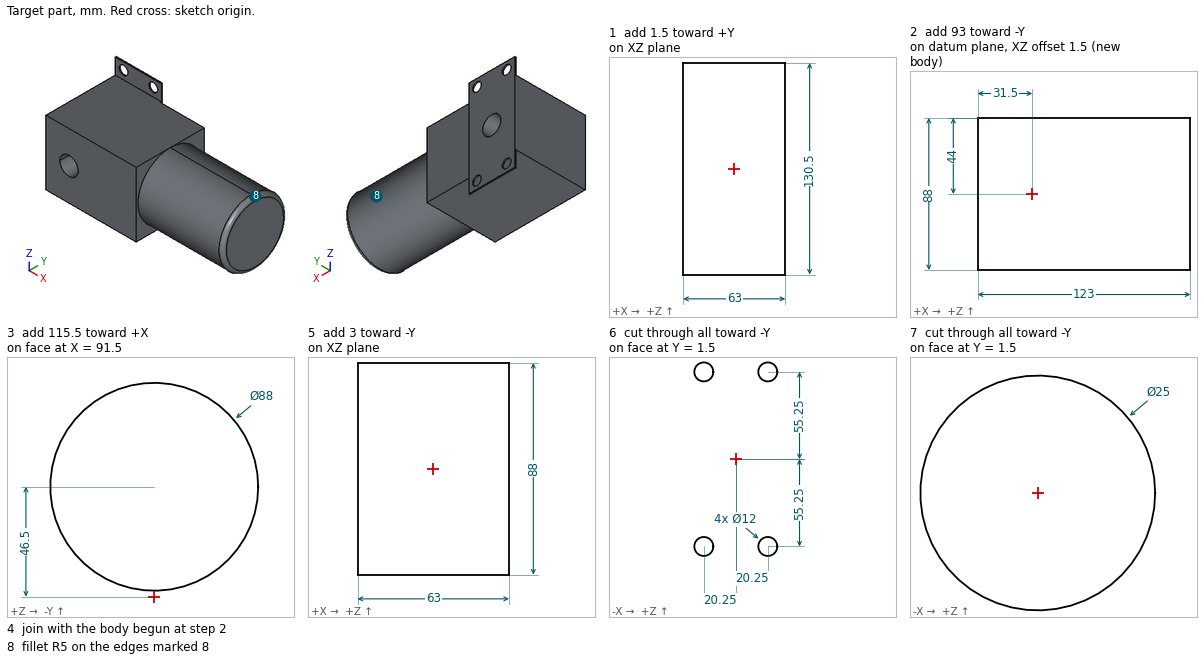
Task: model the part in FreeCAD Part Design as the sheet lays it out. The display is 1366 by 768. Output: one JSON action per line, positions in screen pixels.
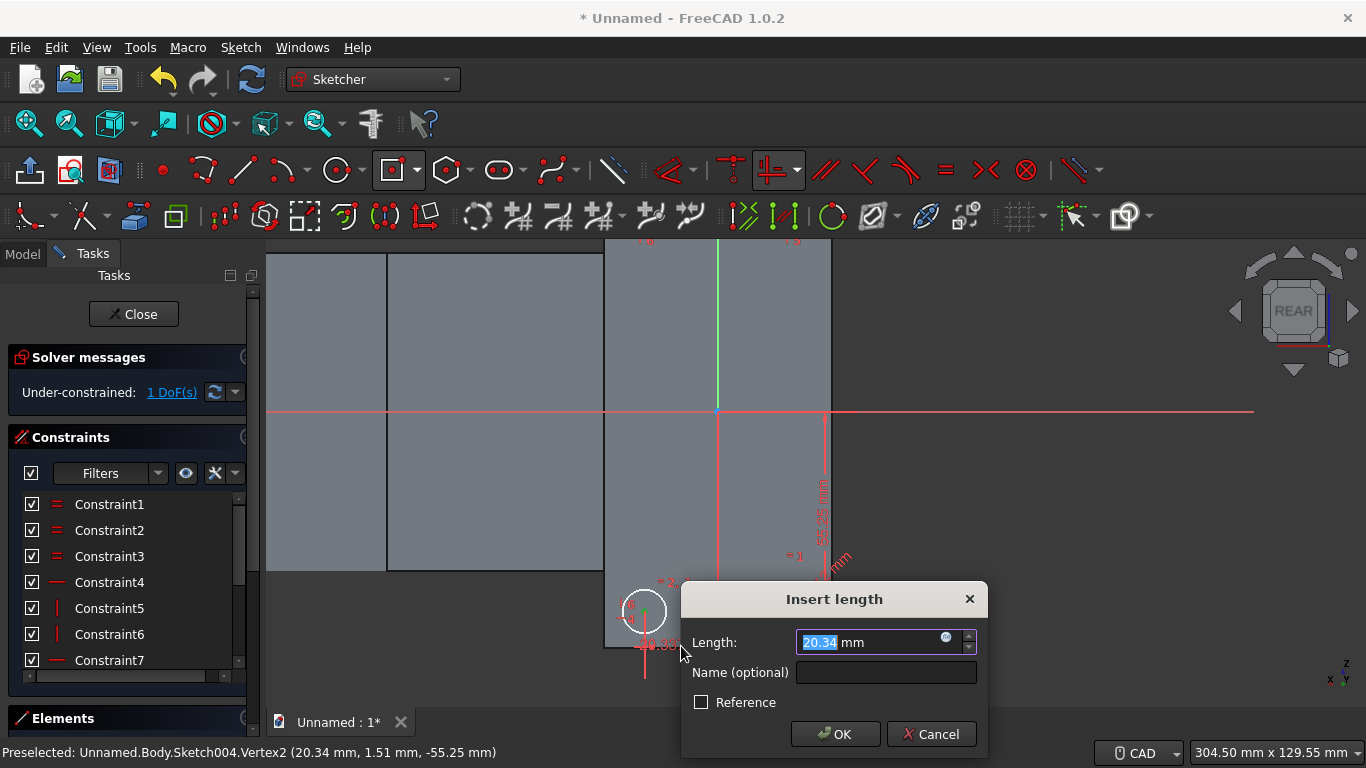
{"action": "type", "text": "20.25"}
{"action": "key", "text": "Return"}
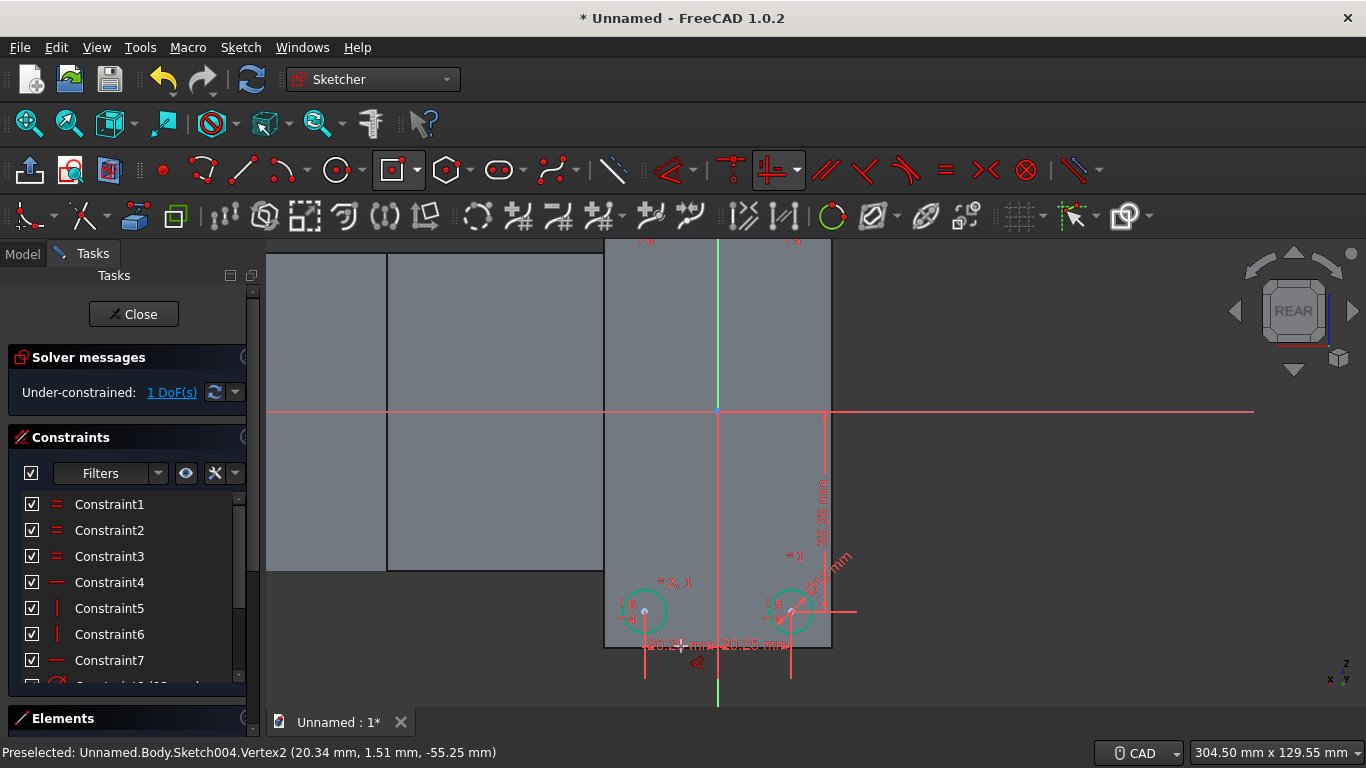
{"action": "scroll", "coordinate": [808, 597], "scroll_direction": "down", "scroll_amount": 2}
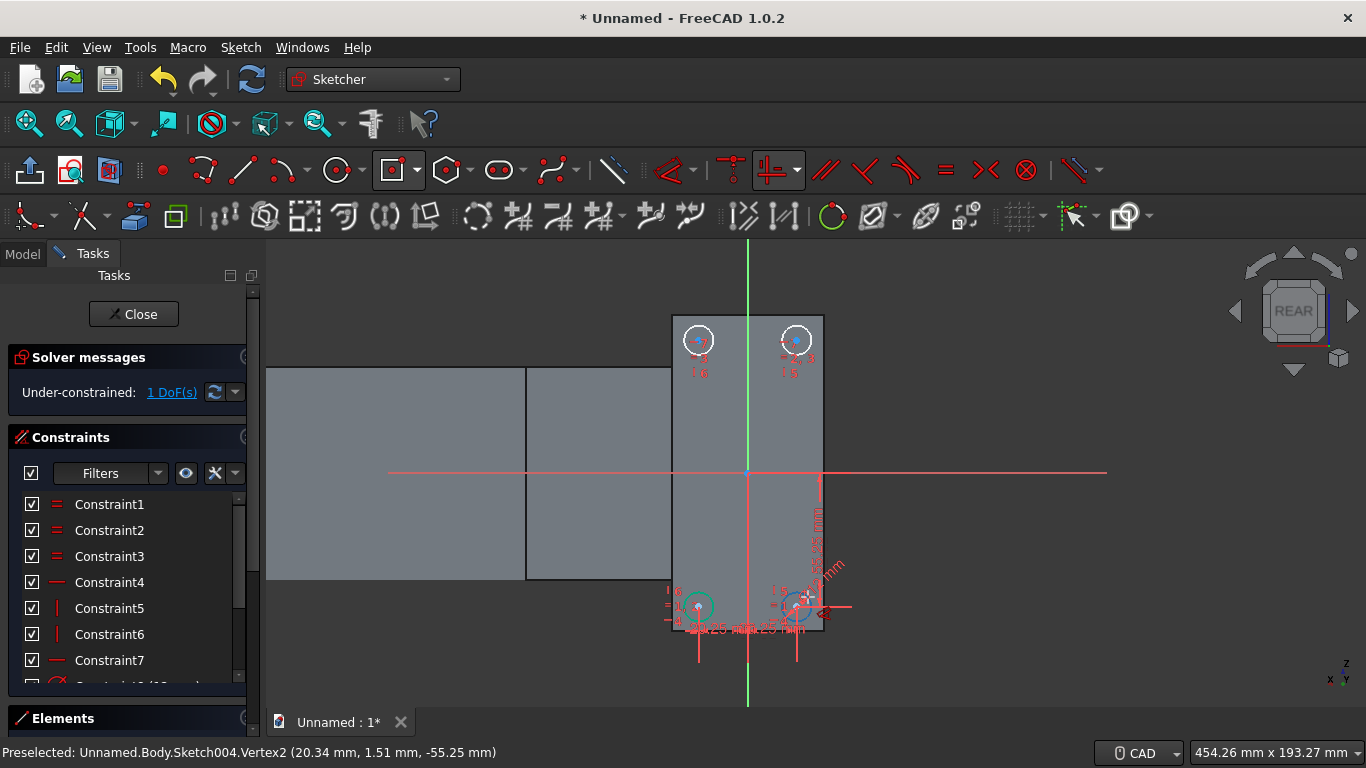
{"action": "left_click", "coordinate": [797, 340]}
{"action": "left_click", "coordinate": [831, 407]}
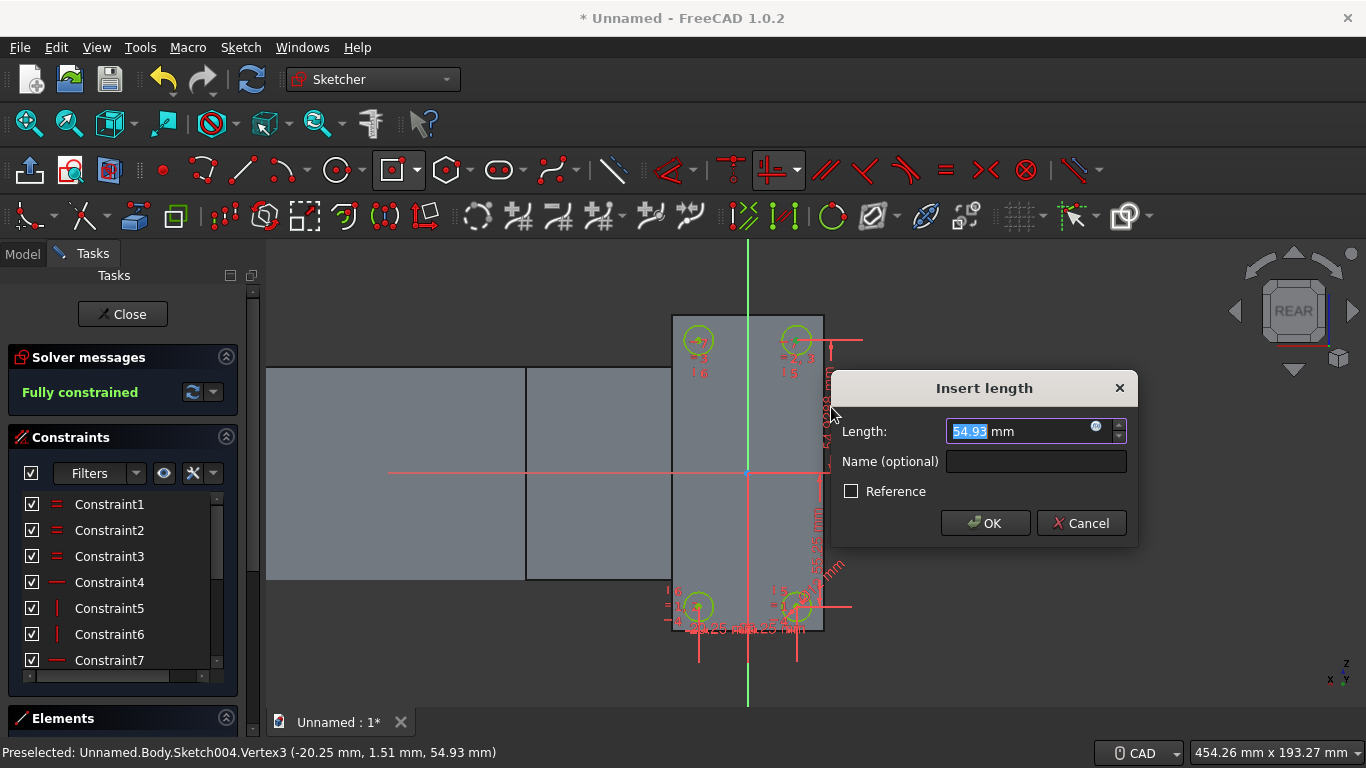
{"action": "type", "text": "55.25"}
{"action": "key", "text": "Return"}
{"action": "key", "text": "Escape"}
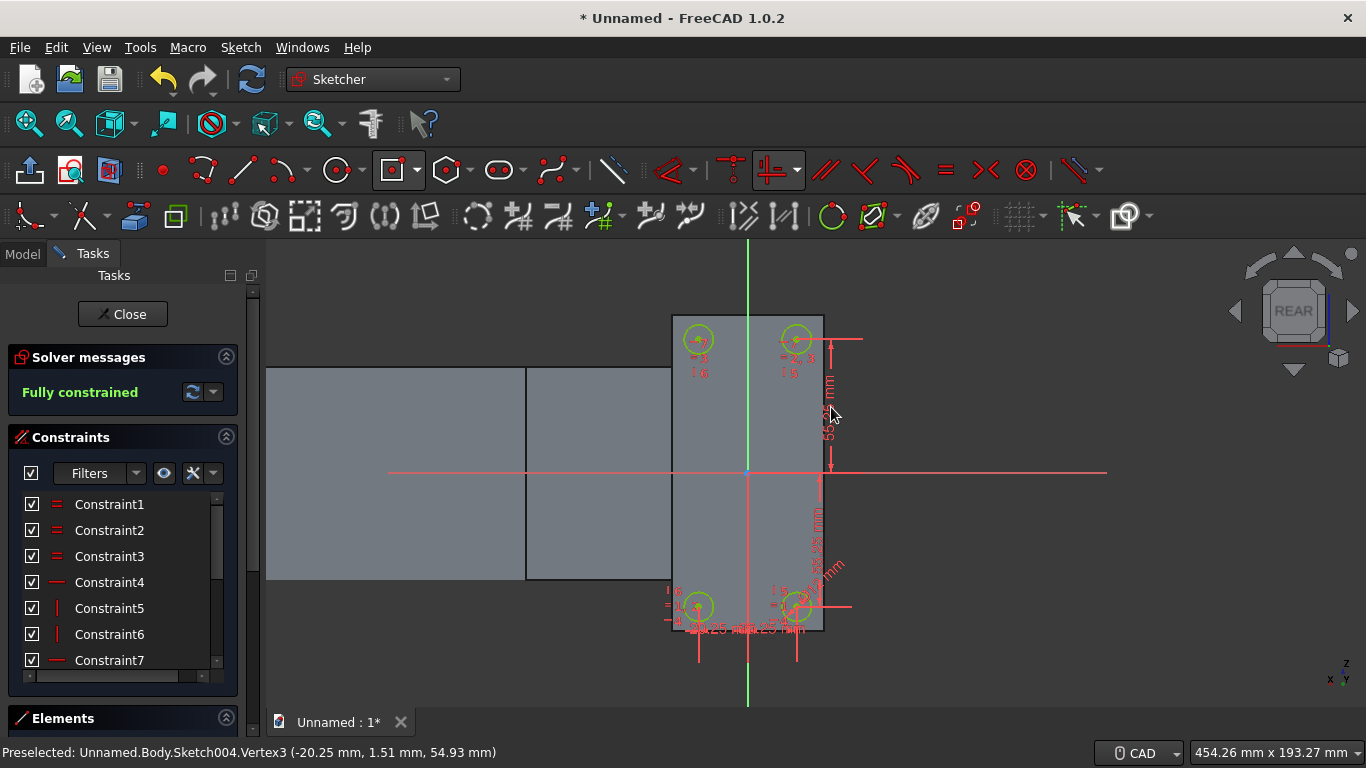
{"action": "left_click", "coordinate": [123, 314]}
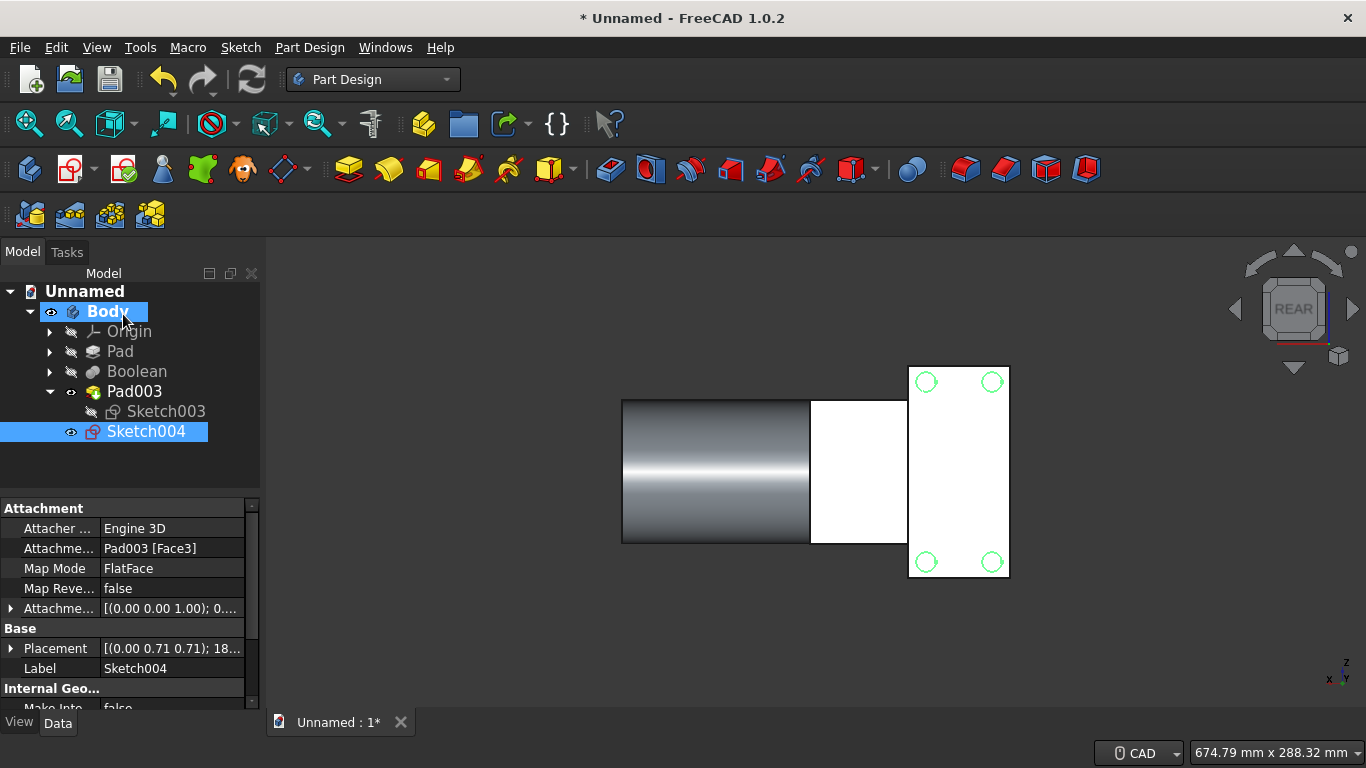
{"action": "left_click", "coordinate": [612, 170]}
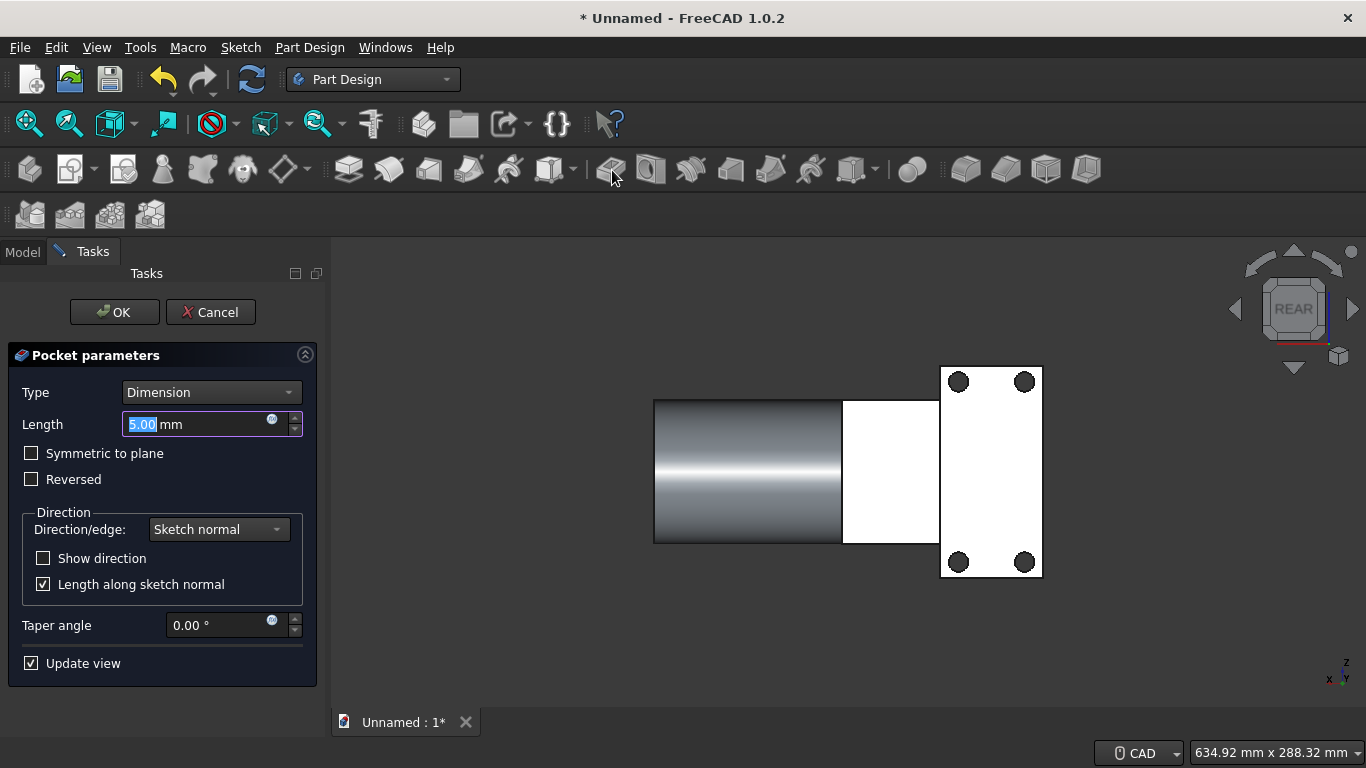
{"action": "left_click", "coordinate": [212, 392]}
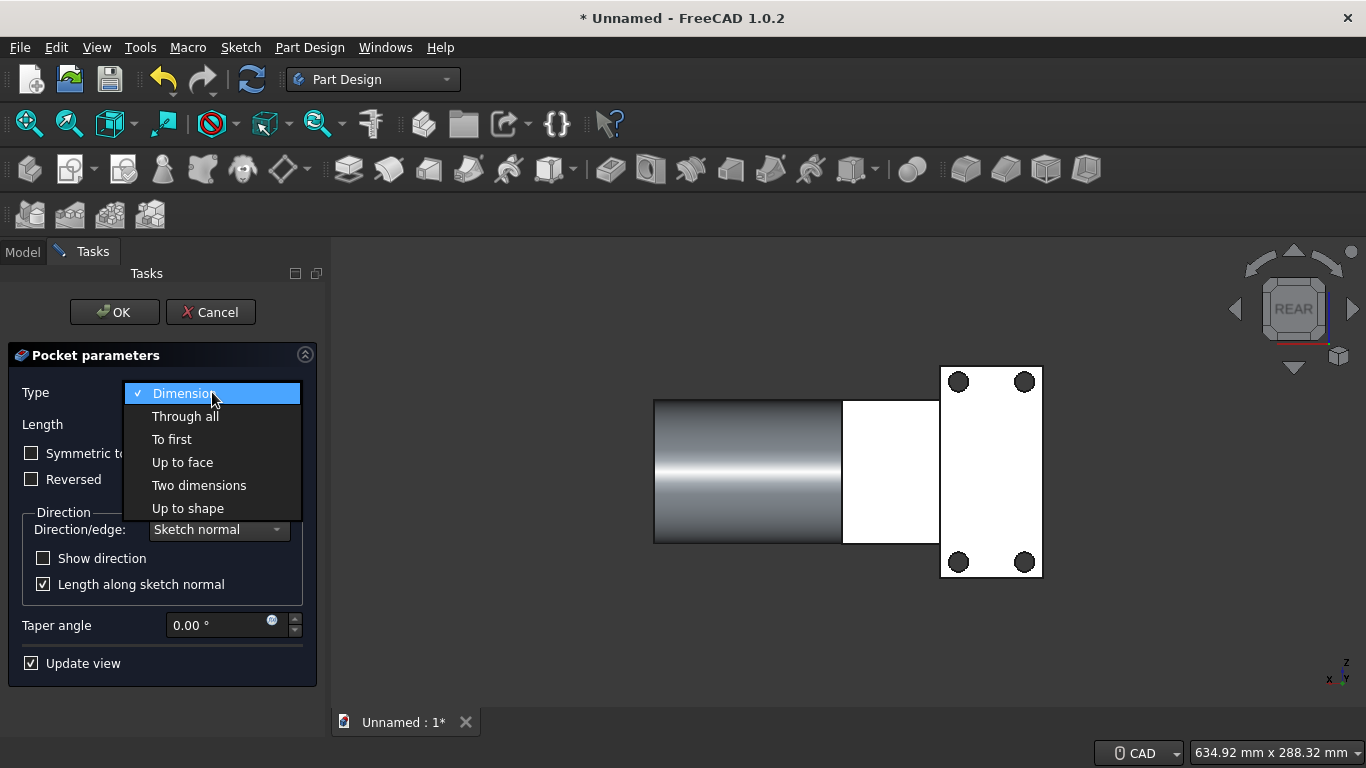
{"action": "left_click", "coordinate": [212, 416]}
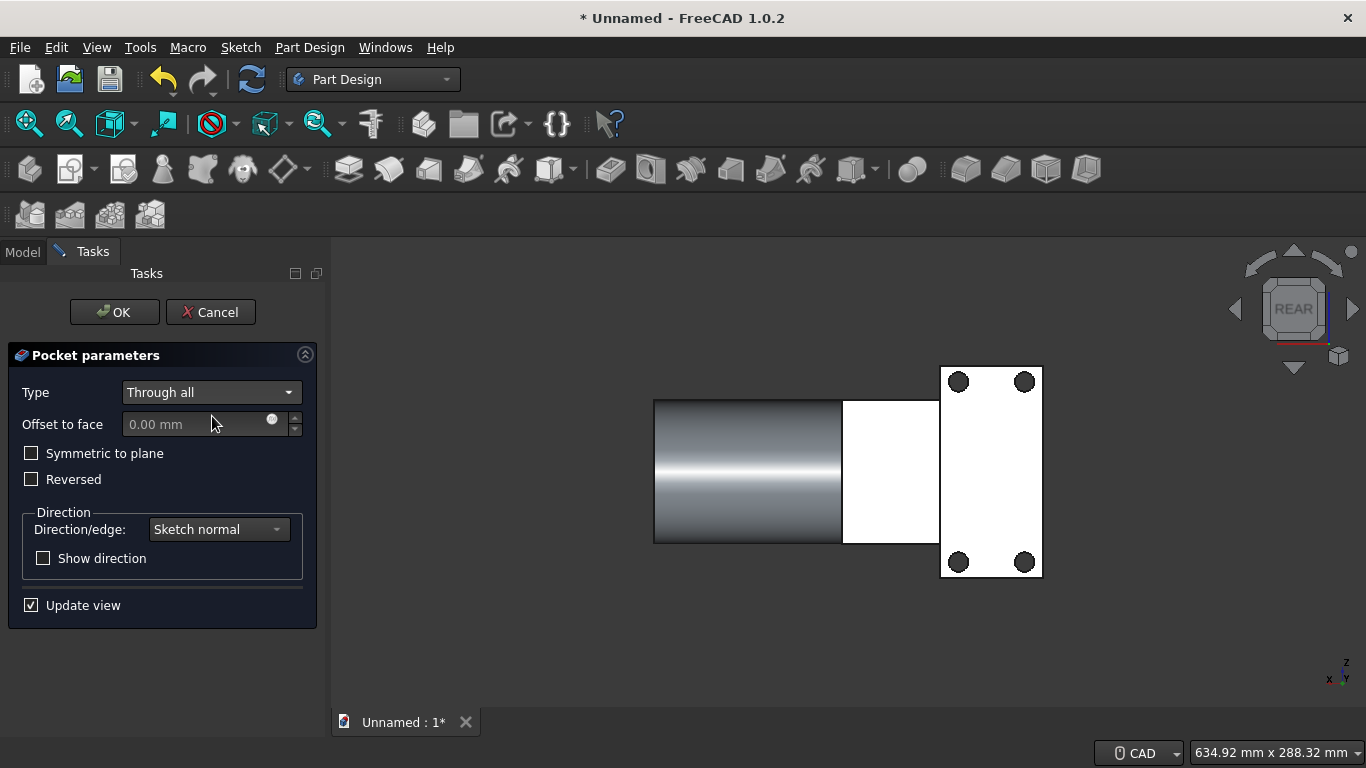
{"action": "left_click", "coordinate": [115, 312]}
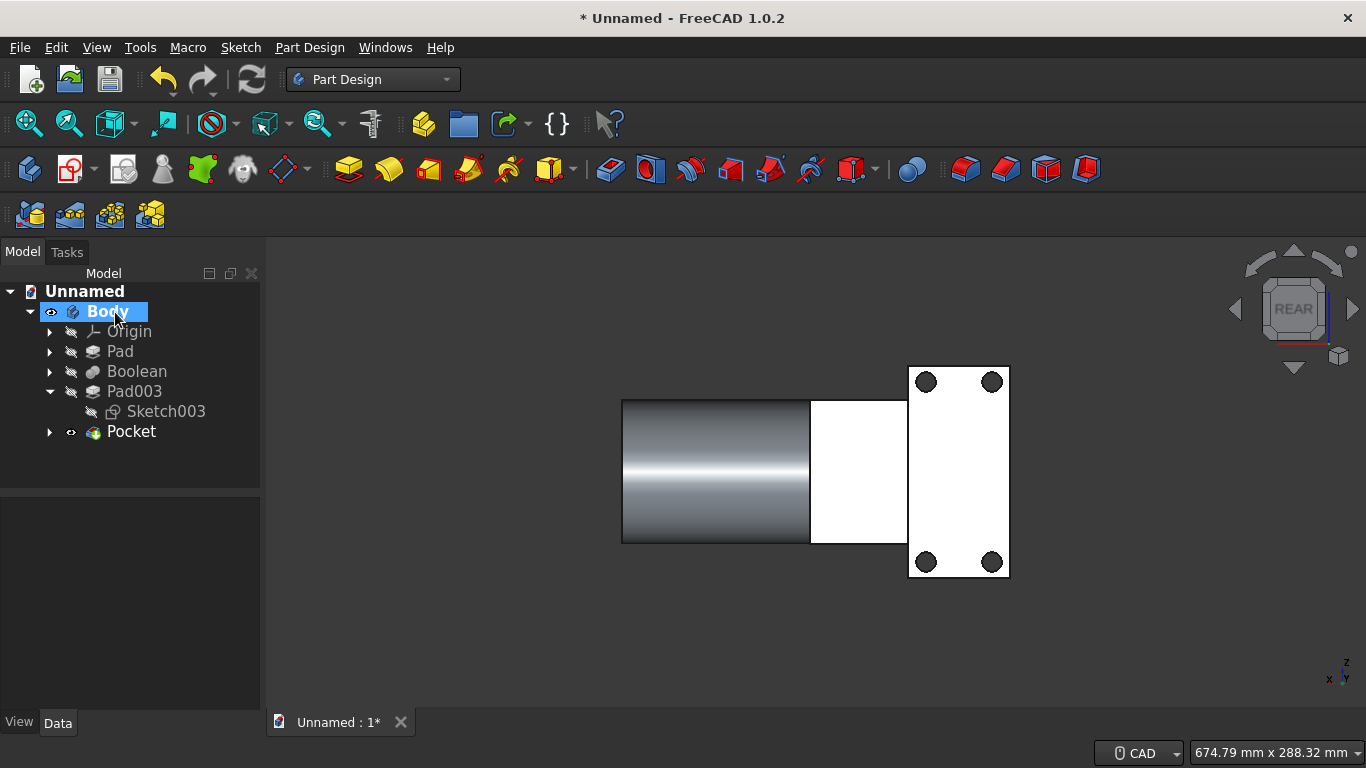
{"action": "left_click", "coordinate": [959, 441]}